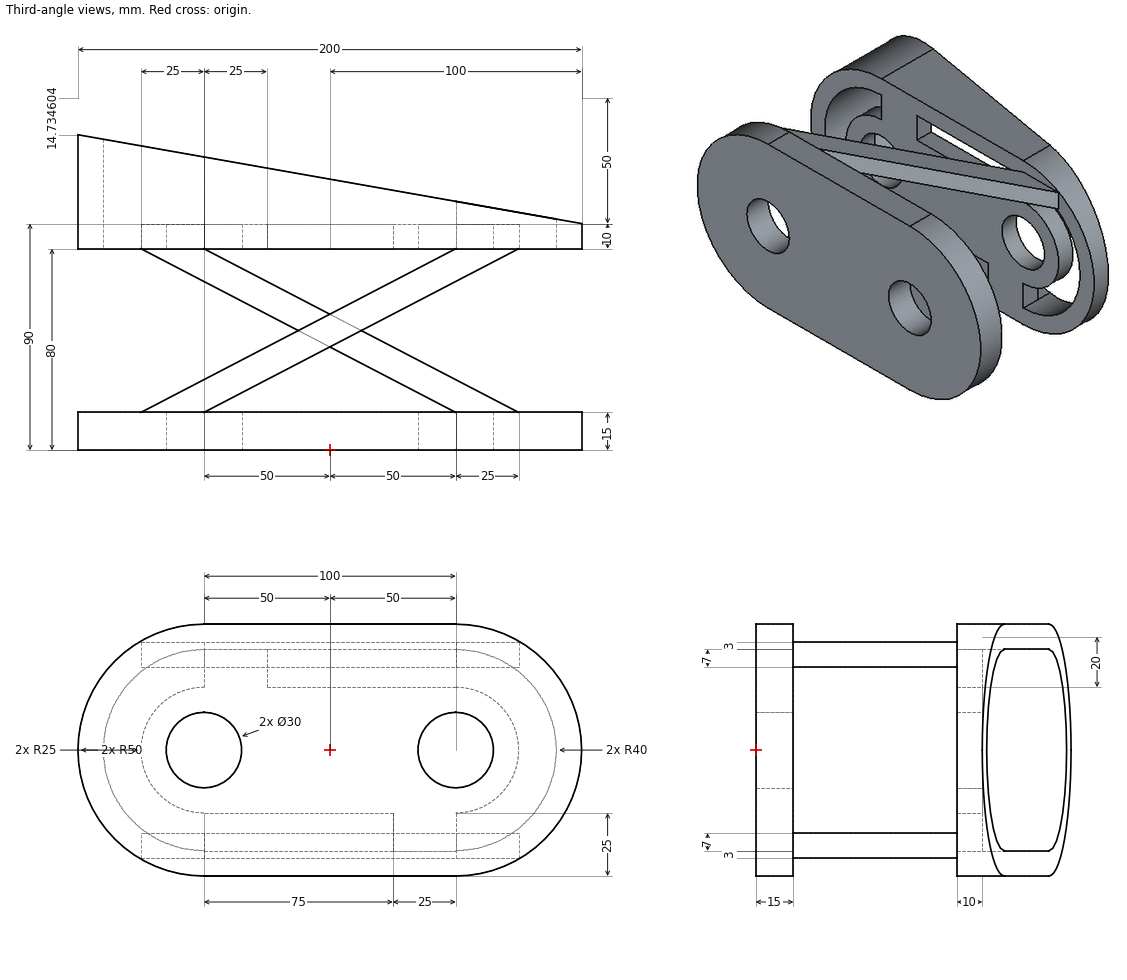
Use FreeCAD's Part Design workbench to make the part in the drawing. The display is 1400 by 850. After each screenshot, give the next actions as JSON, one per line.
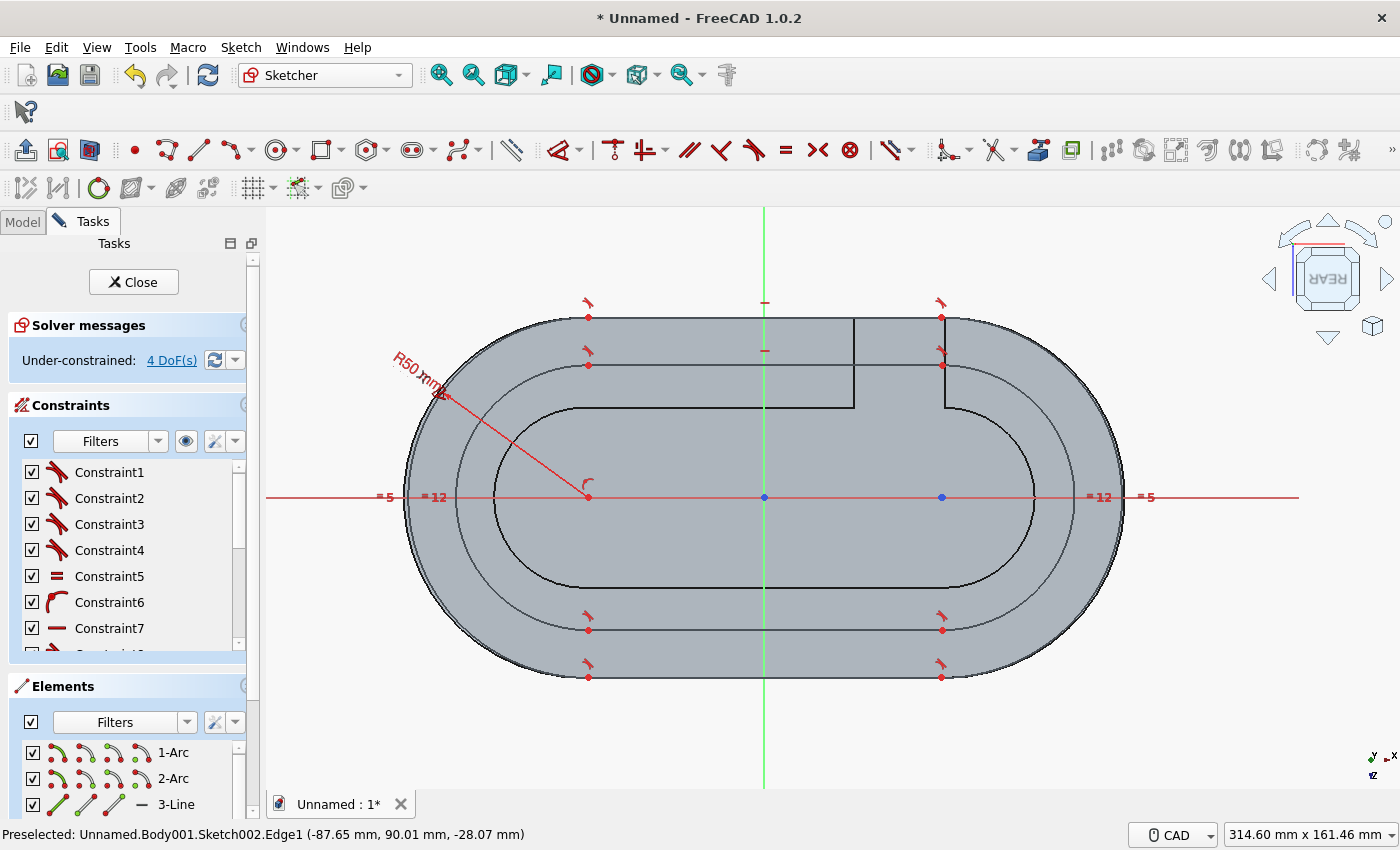
{"action": "left_click", "coordinate": [481, 420]}
{"action": "left_click", "coordinate": [455, 401]}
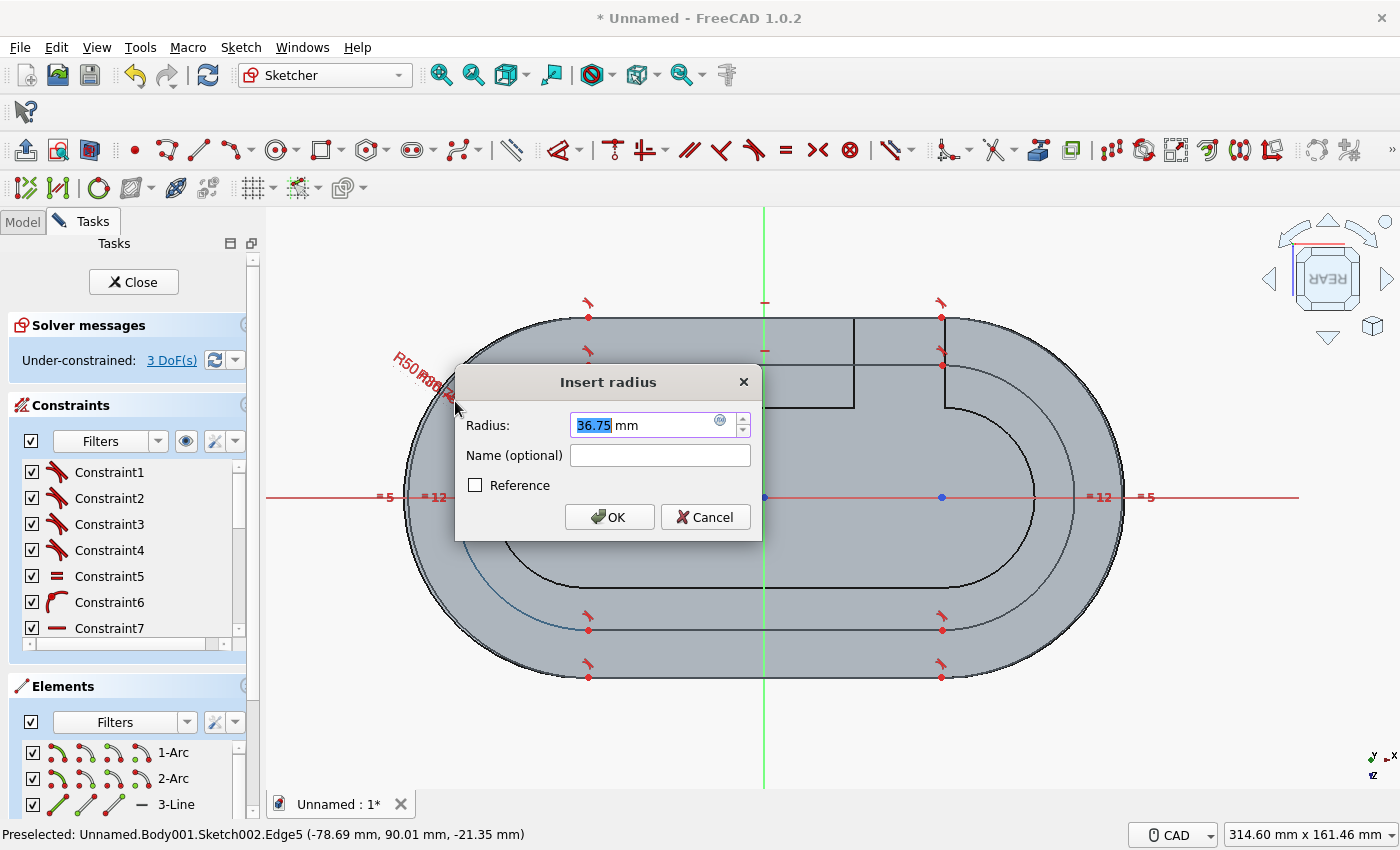
{"action": "type", "text": "40"}
{"action": "key", "text": "Return"}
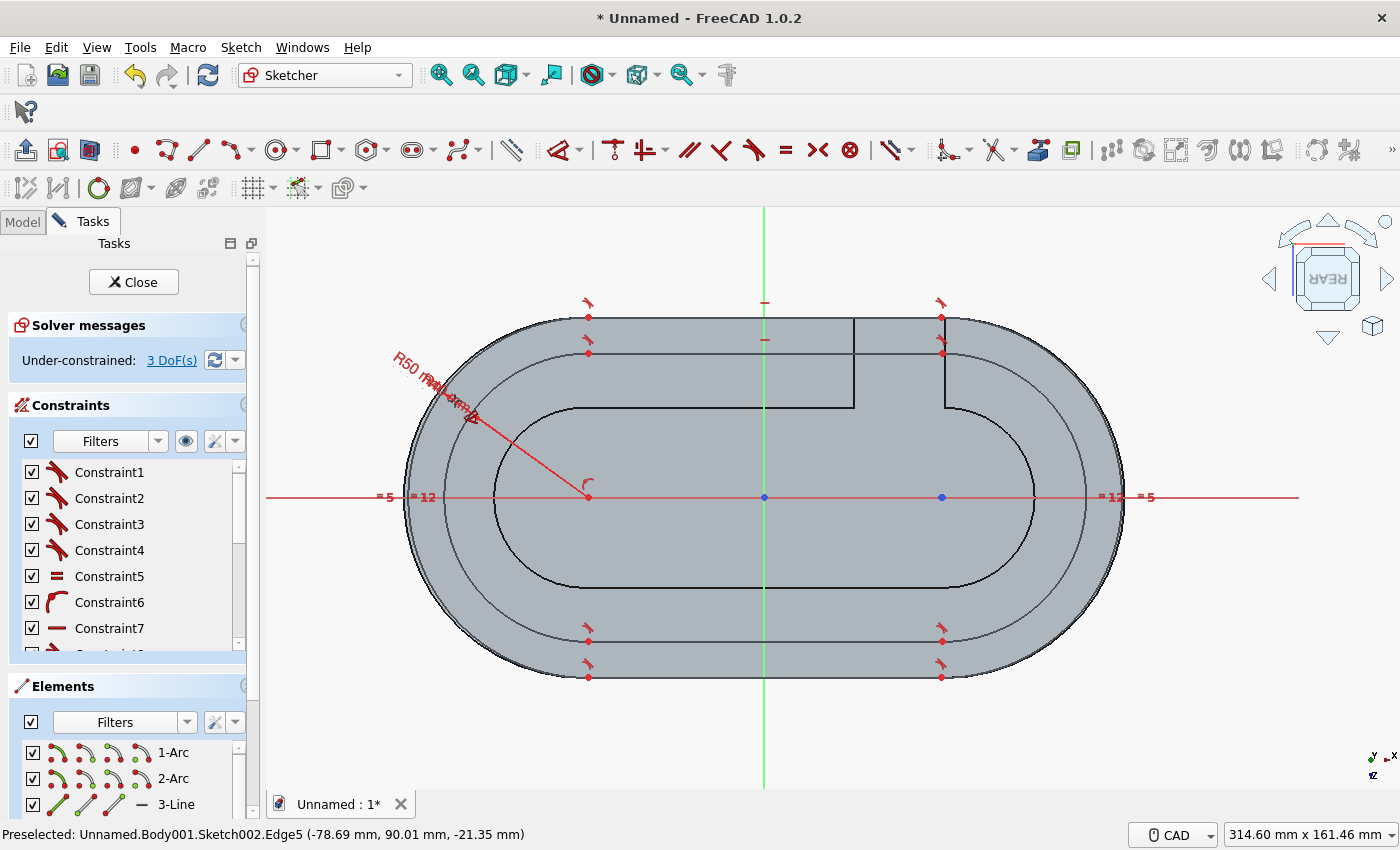
{"action": "left_click", "coordinate": [694, 318]}
{"action": "left_click", "coordinate": [684, 284]}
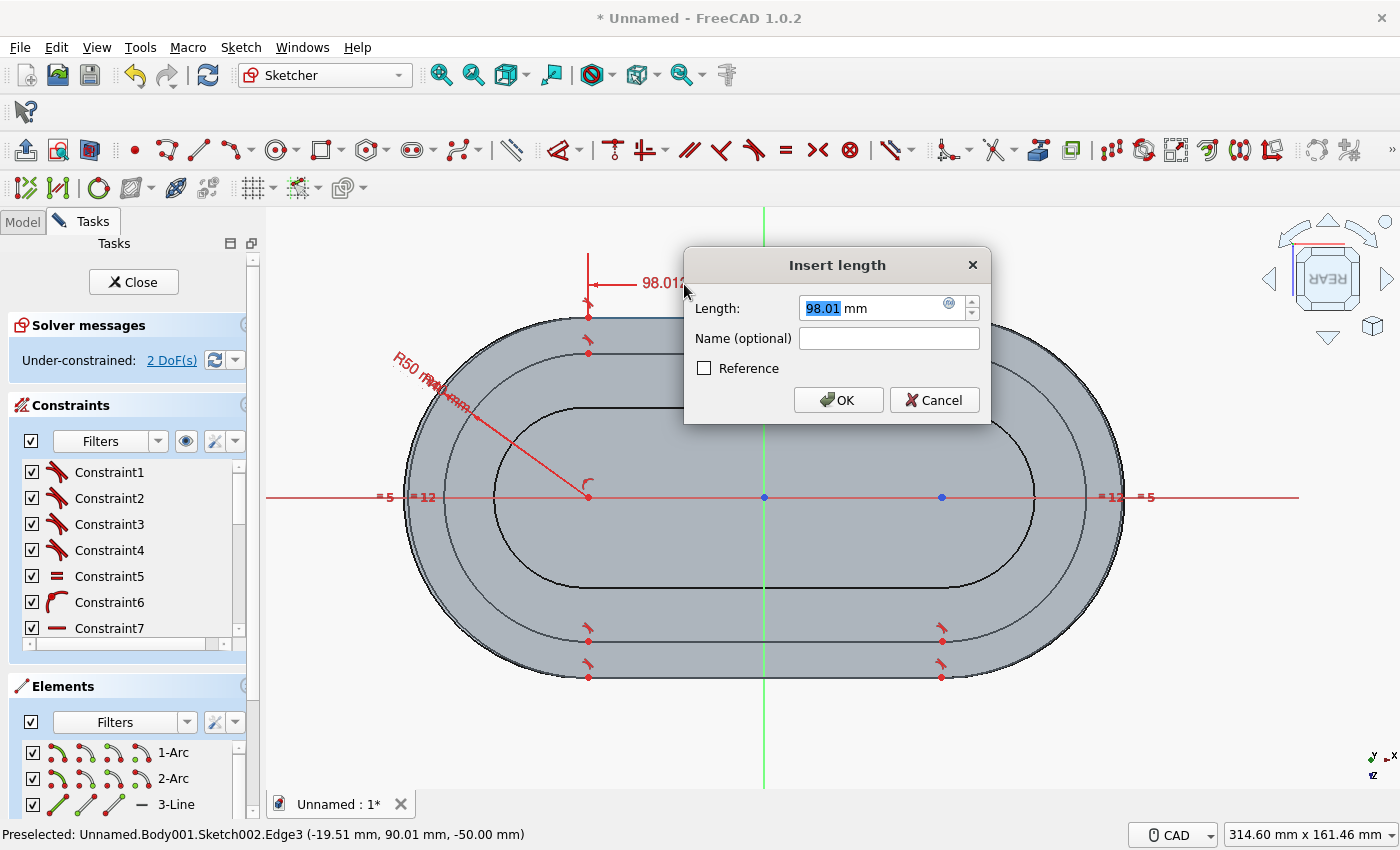
{"action": "type", "text": "100"}
{"action": "key", "text": "Return"}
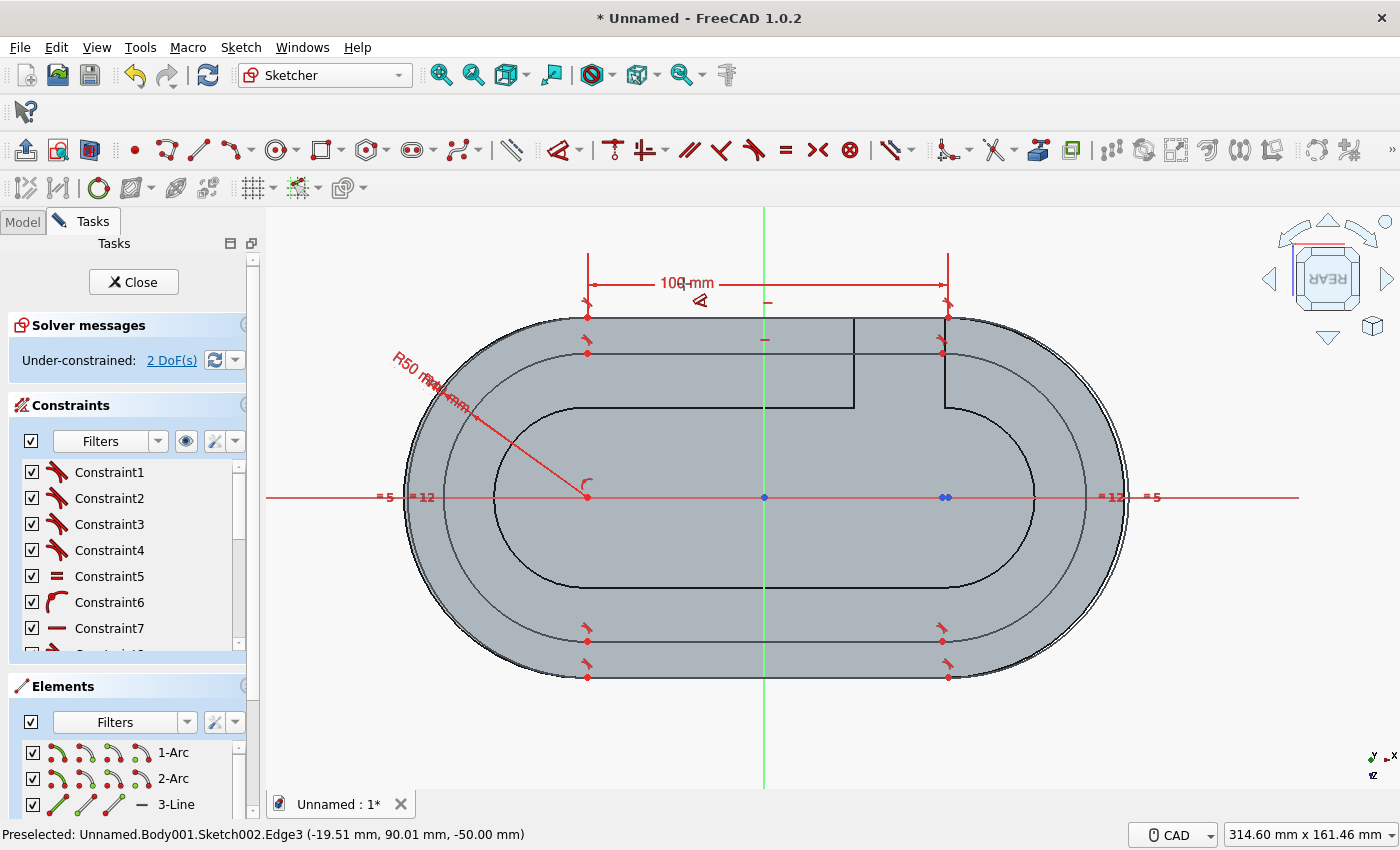
{"action": "left_click", "coordinate": [694, 354]}
{"action": "left_click", "coordinate": [684, 388]}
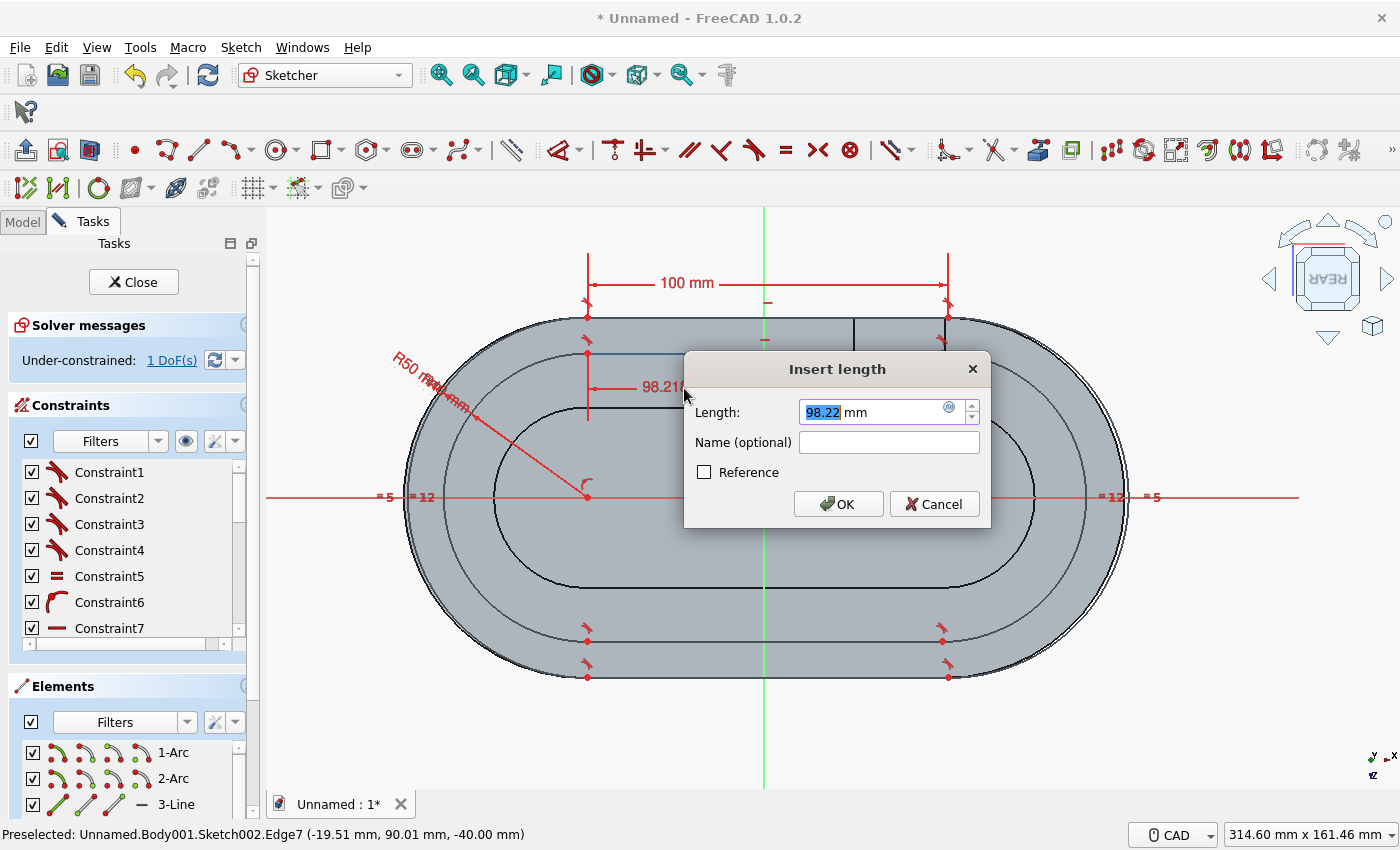
{"action": "type", "text": "100"}
{"action": "key", "text": "Return"}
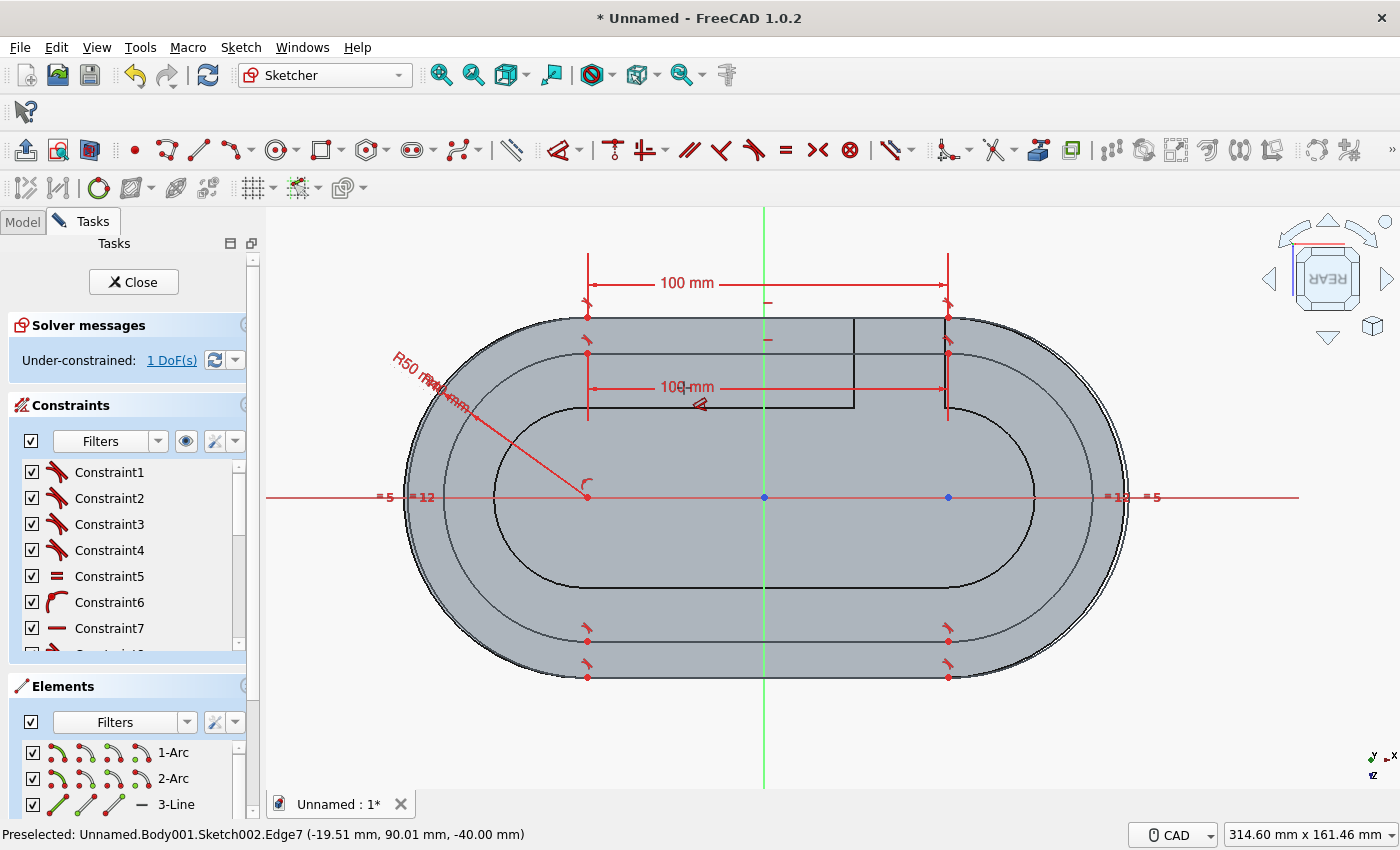
{"action": "left_click", "coordinate": [588, 318]}
{"action": "left_click", "coordinate": [676, 532]}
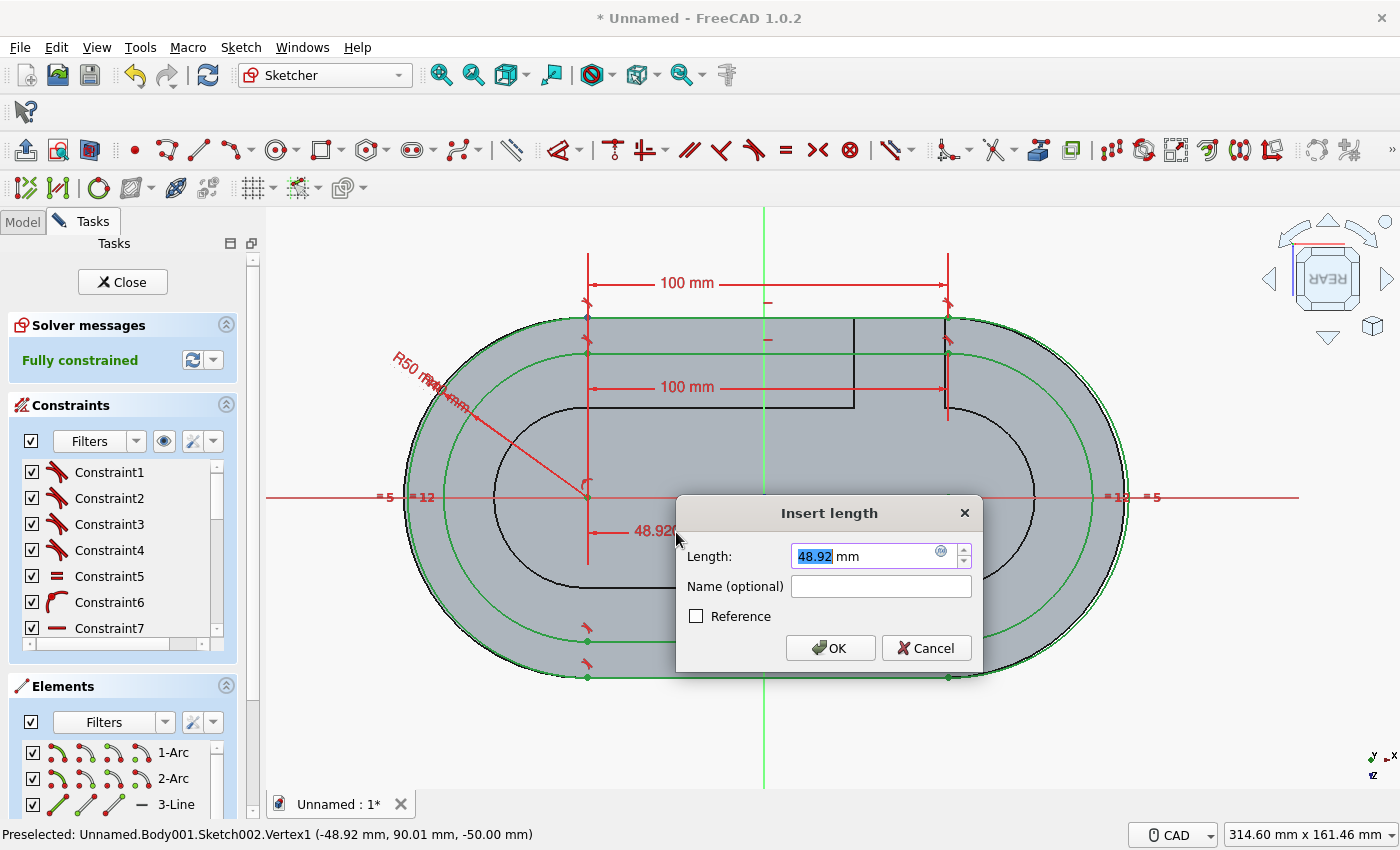
{"action": "type", "text": "50"}
{"action": "key", "text": "Return"}
{"action": "key", "text": "Escape"}